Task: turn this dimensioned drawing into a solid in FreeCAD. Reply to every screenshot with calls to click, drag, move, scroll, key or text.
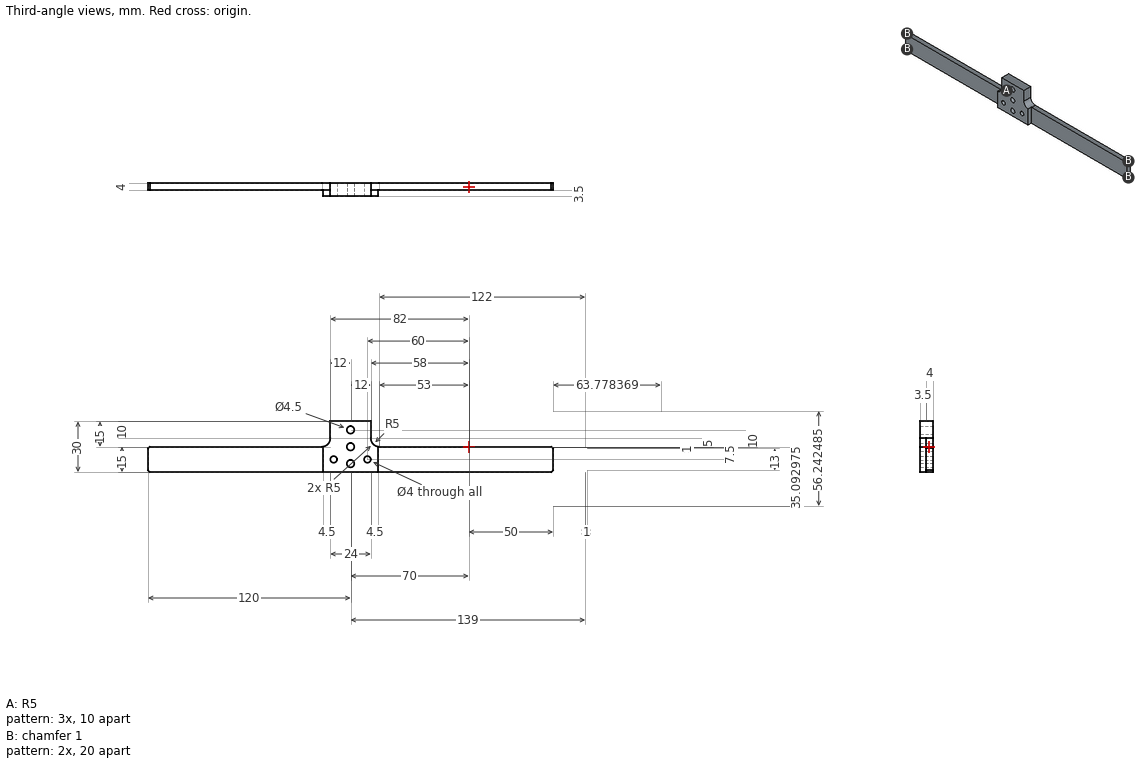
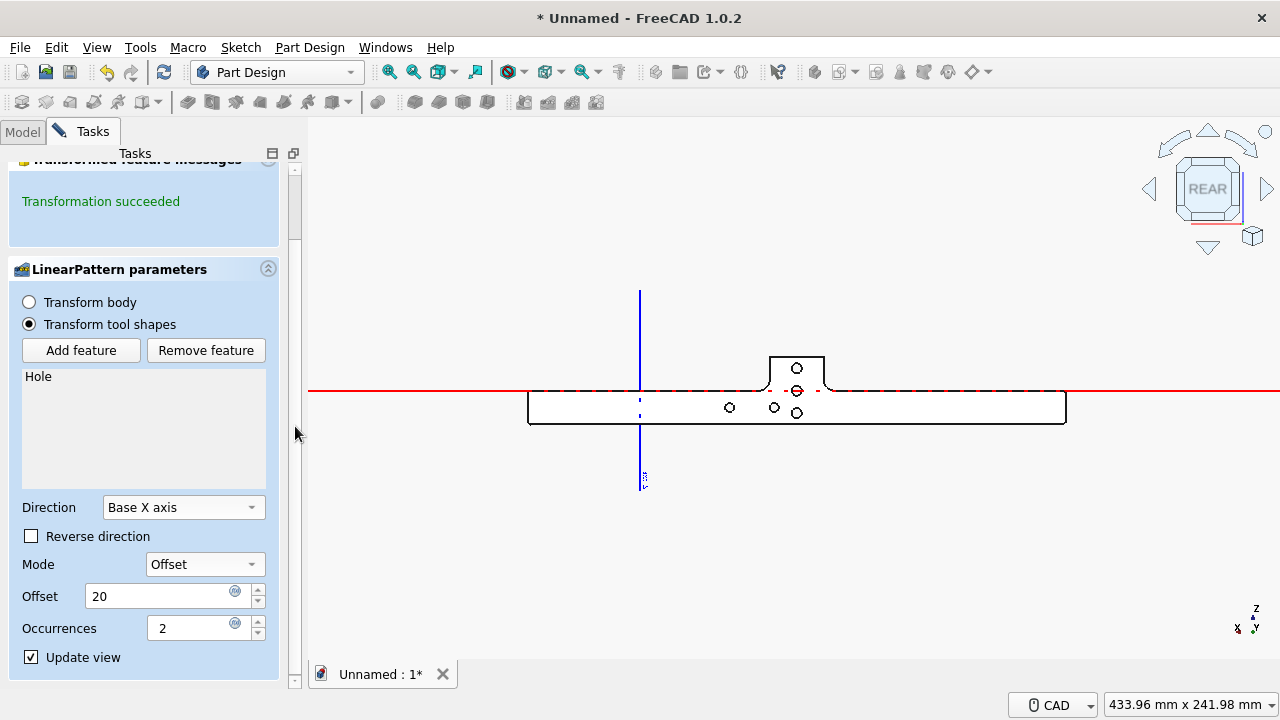
triple_click(198, 628)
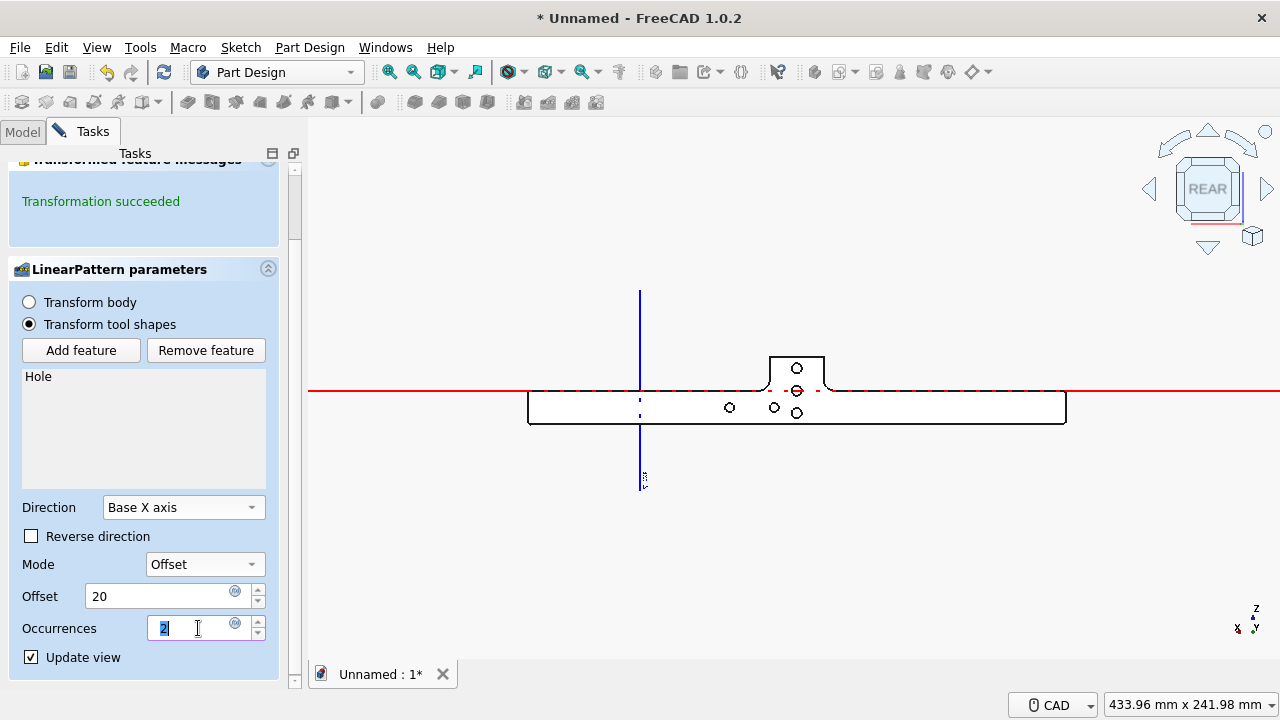
text(2)
key(Tab)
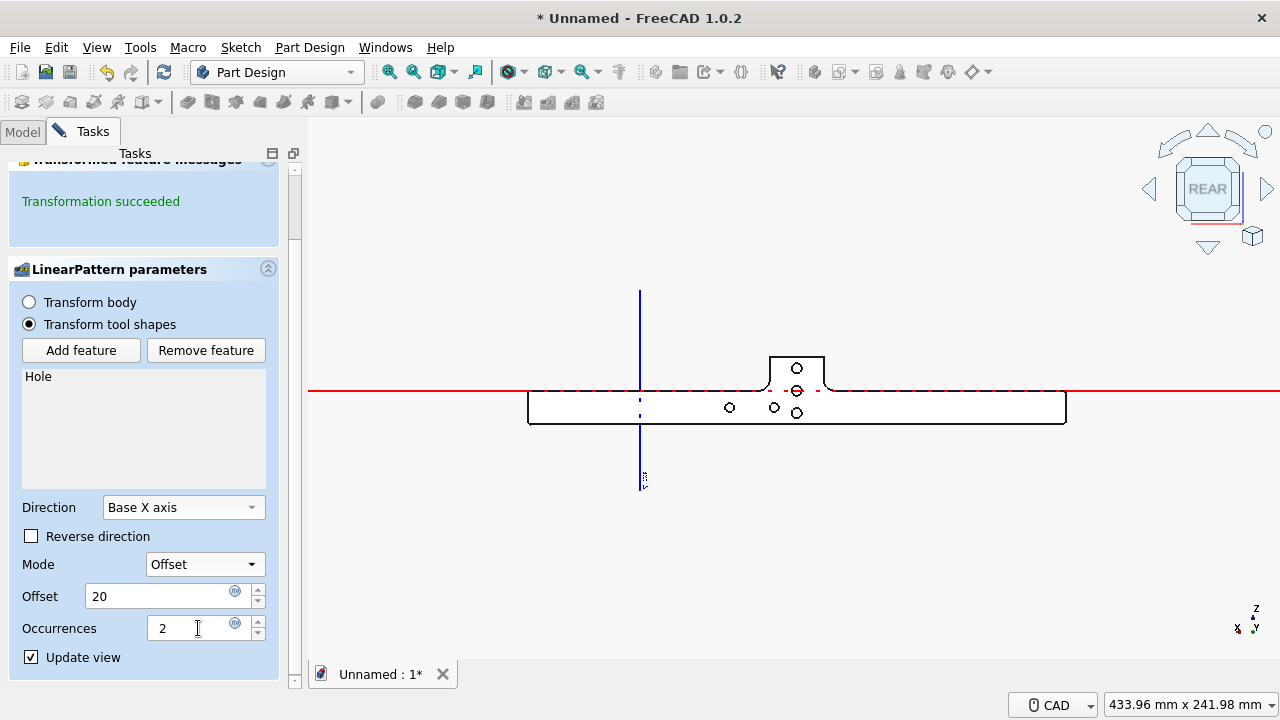
click(30, 536)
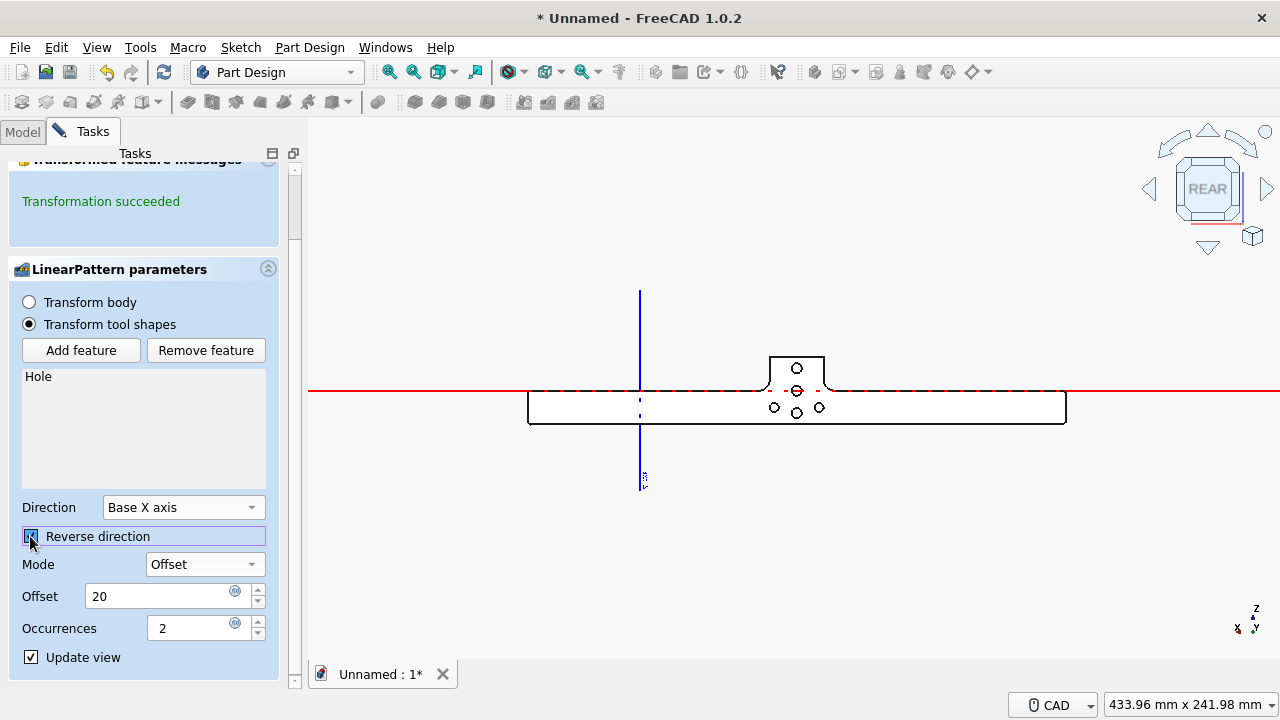
scroll(295, 426, up, 3)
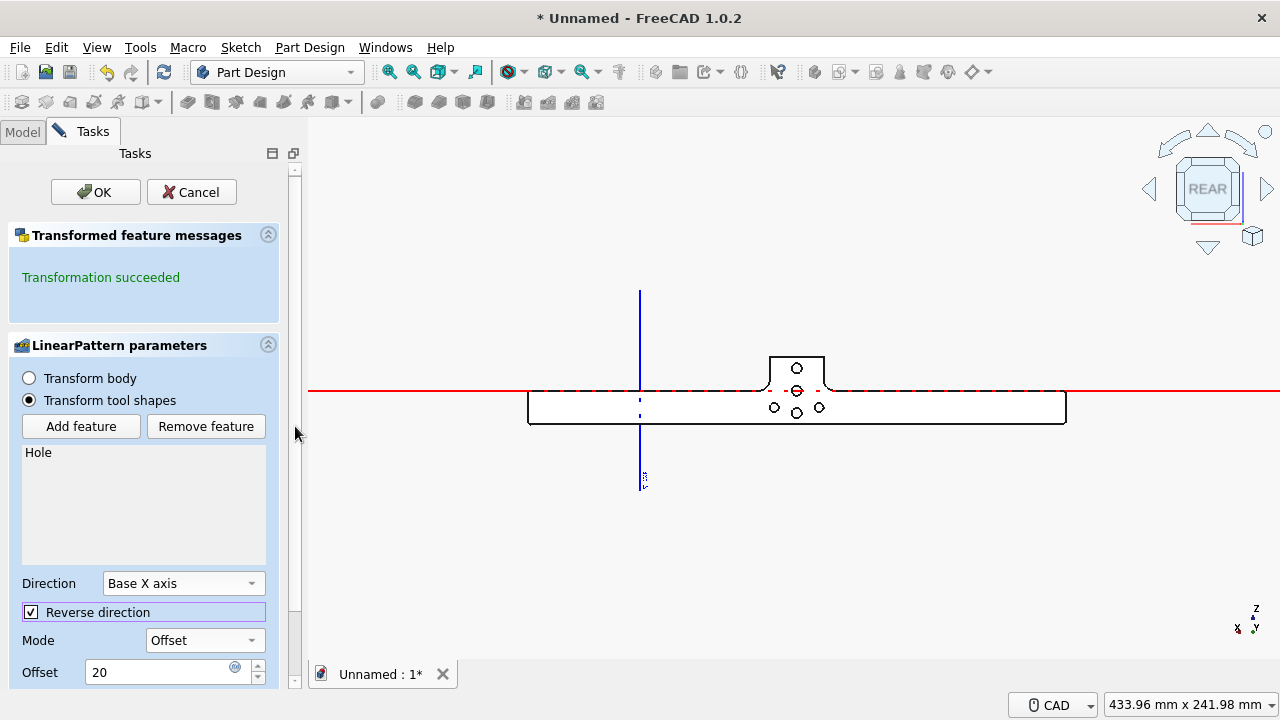
click(96, 192)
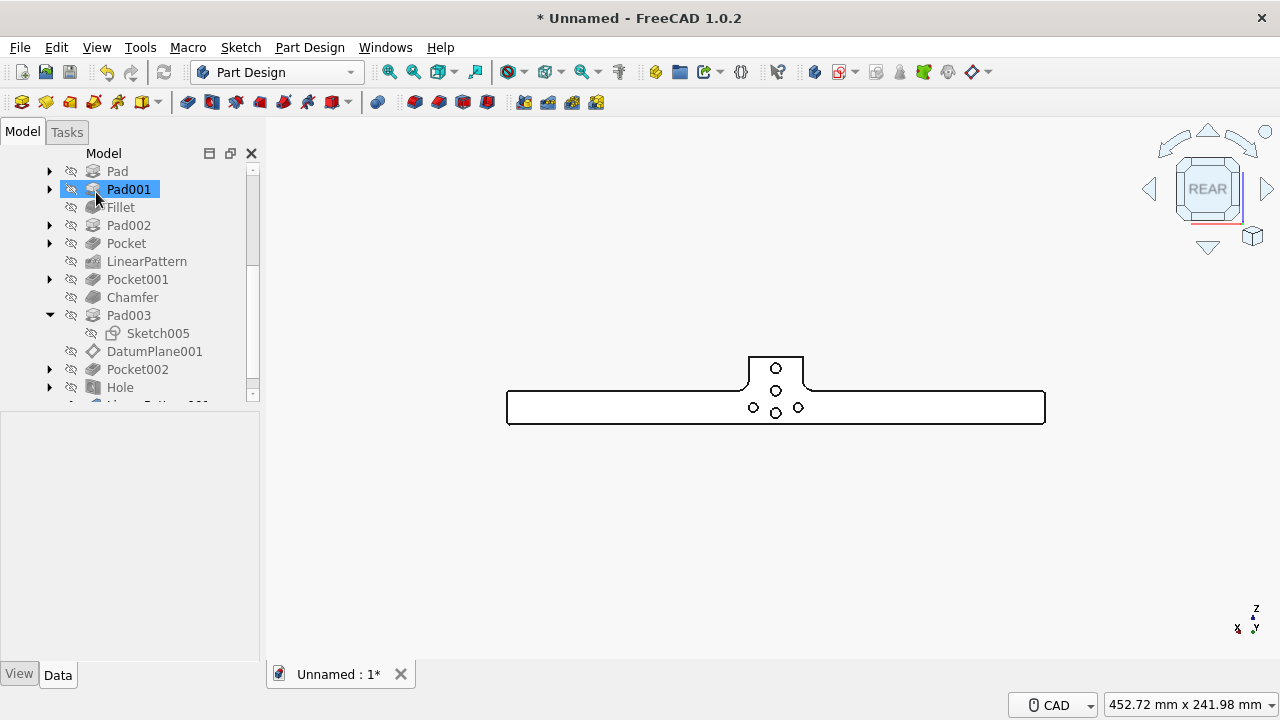
key(0)